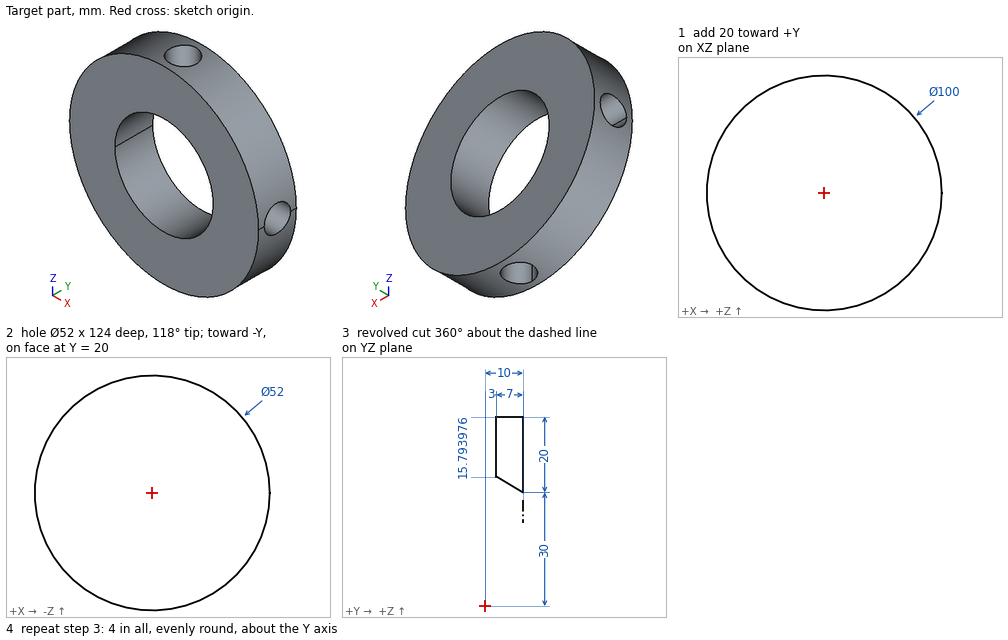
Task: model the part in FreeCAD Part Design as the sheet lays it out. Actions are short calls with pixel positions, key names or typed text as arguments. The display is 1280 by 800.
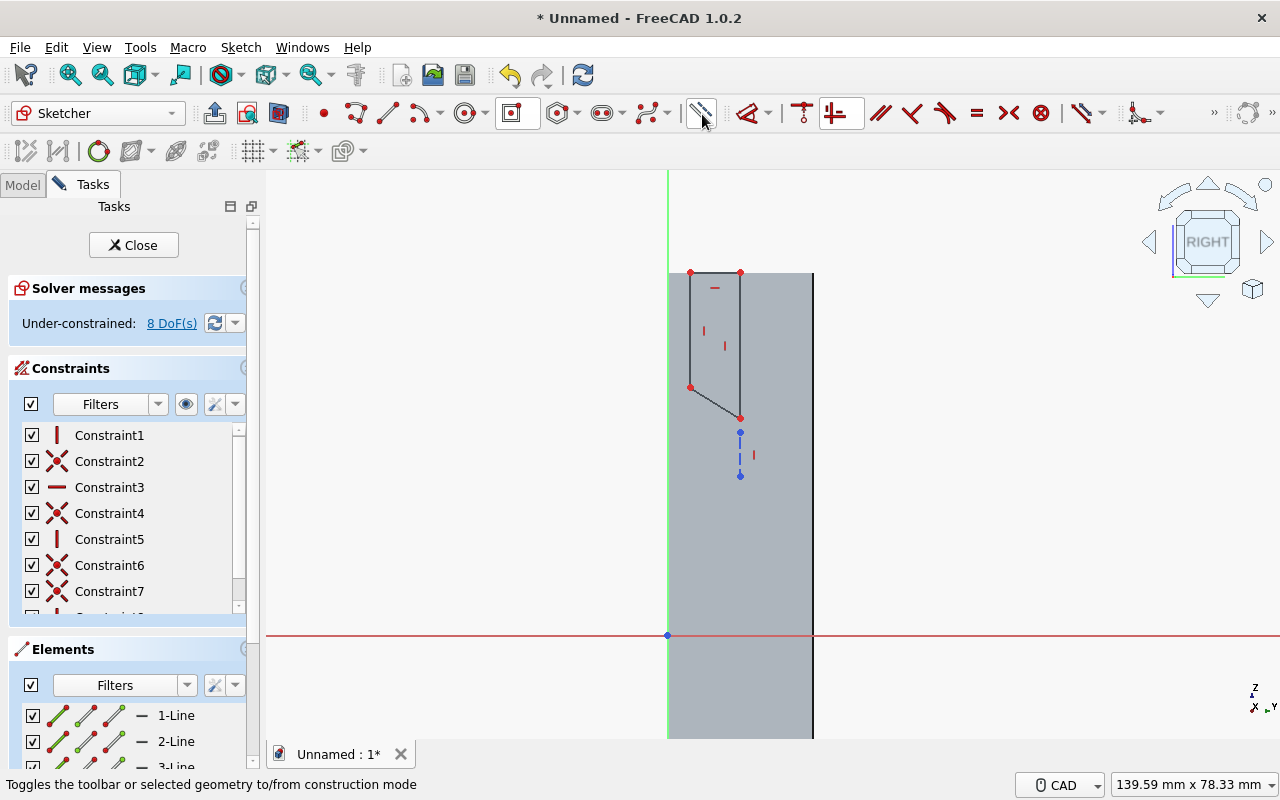
click(725, 273)
click(715, 239)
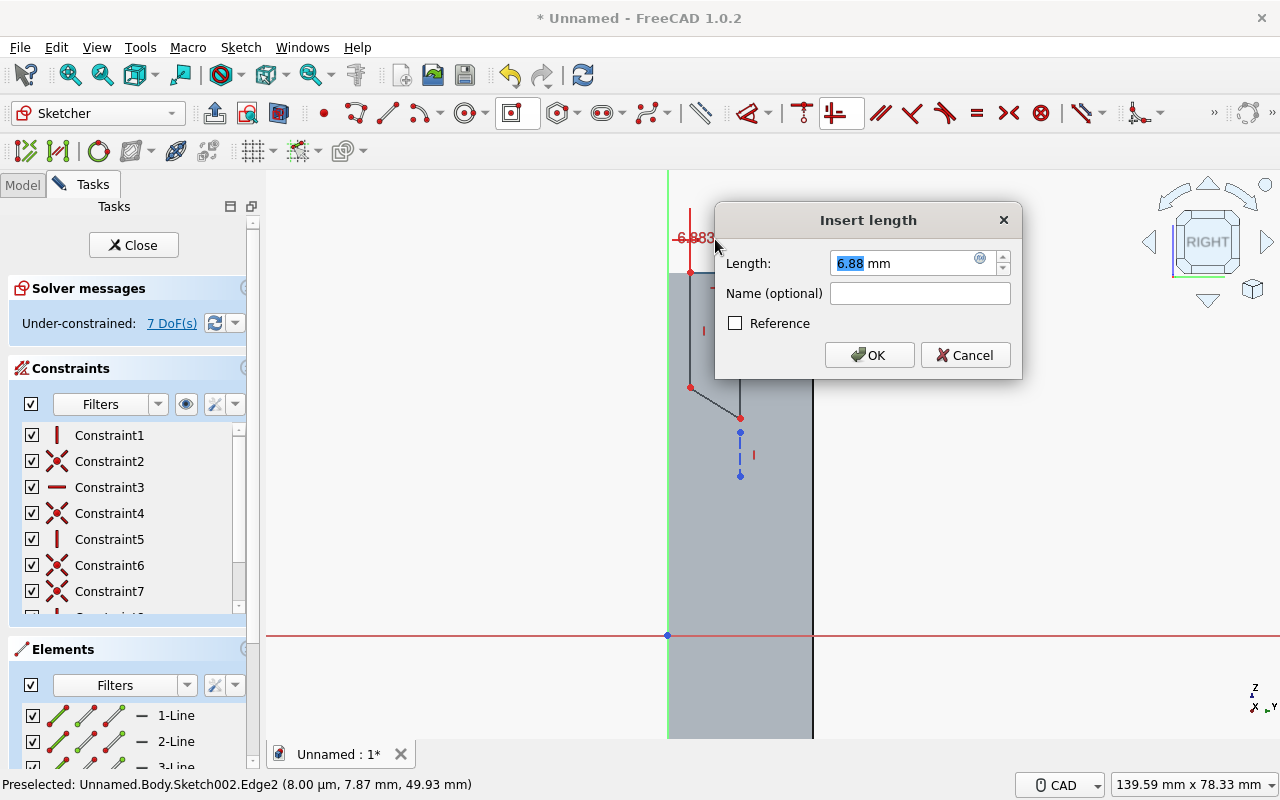
text(7)
key(Return)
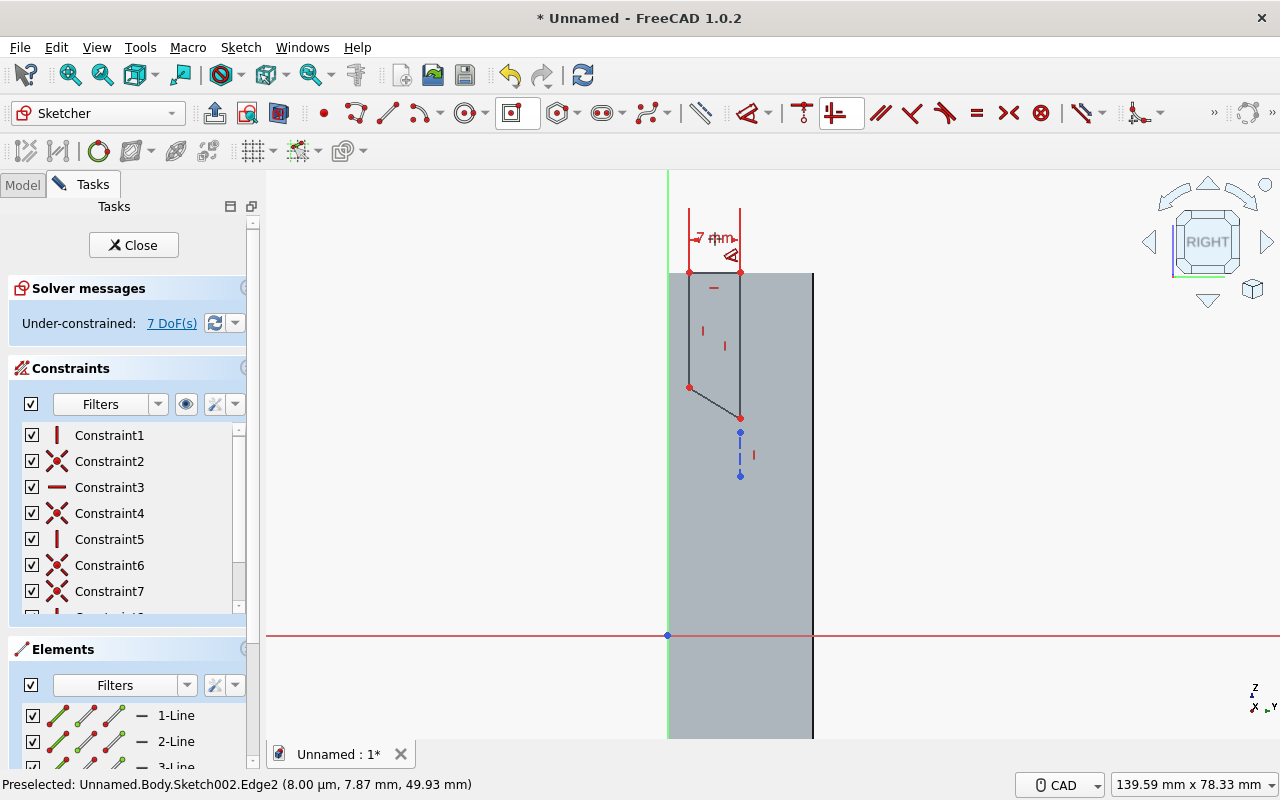
click(740, 375)
click(774, 346)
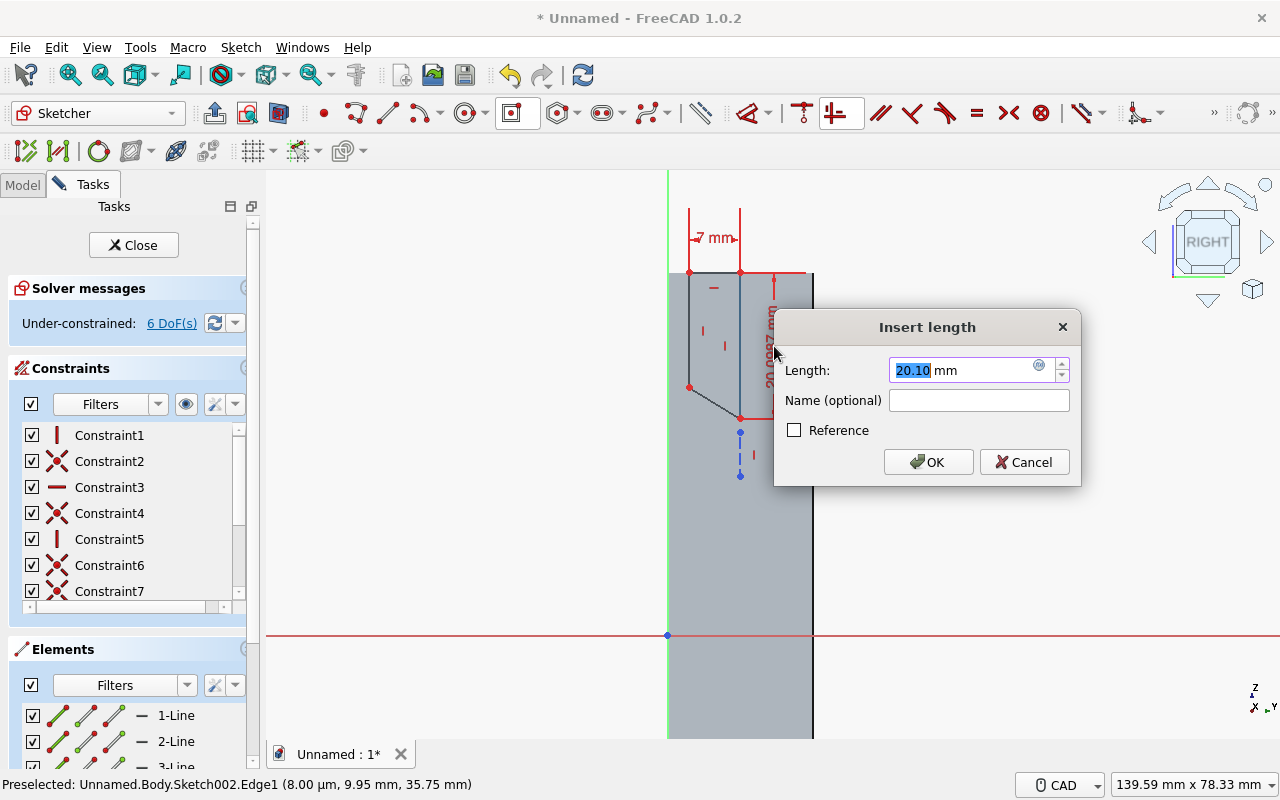
text(20)
key(Return)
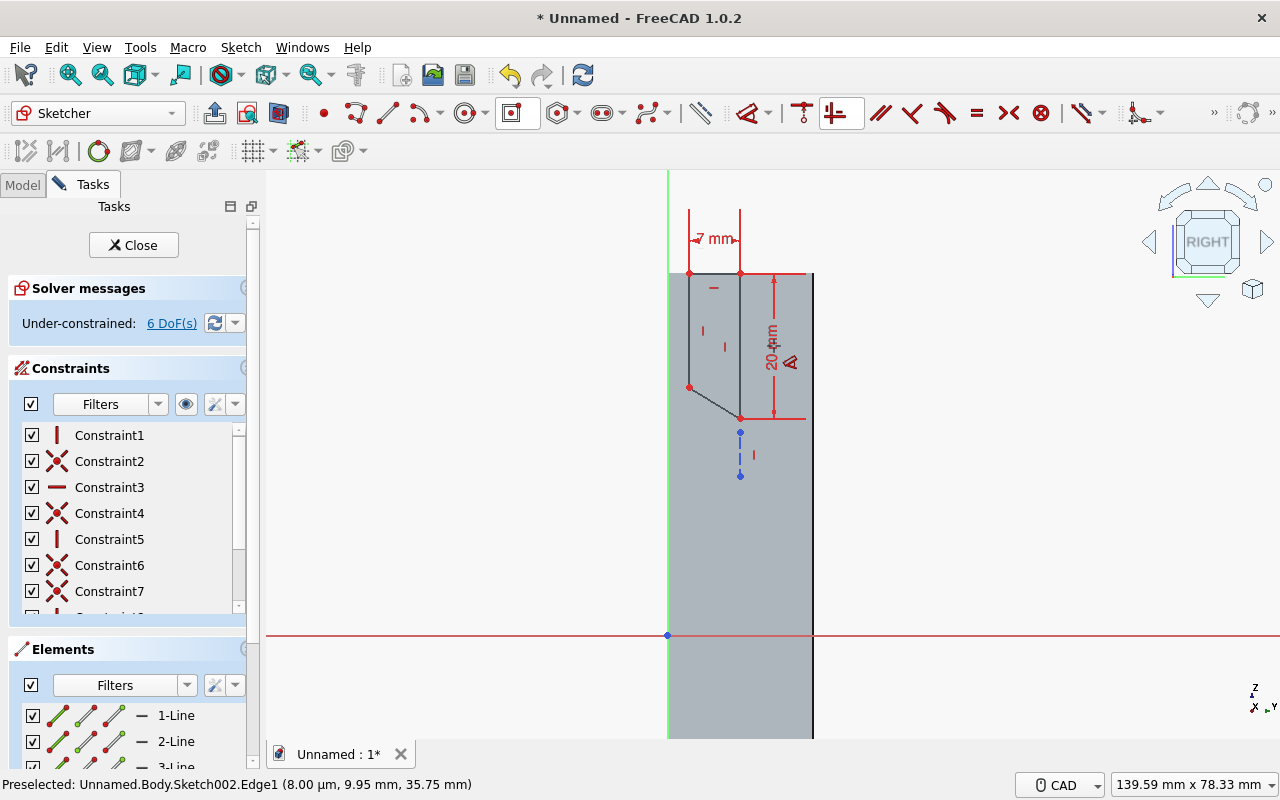
scroll(689, 274, up, 3)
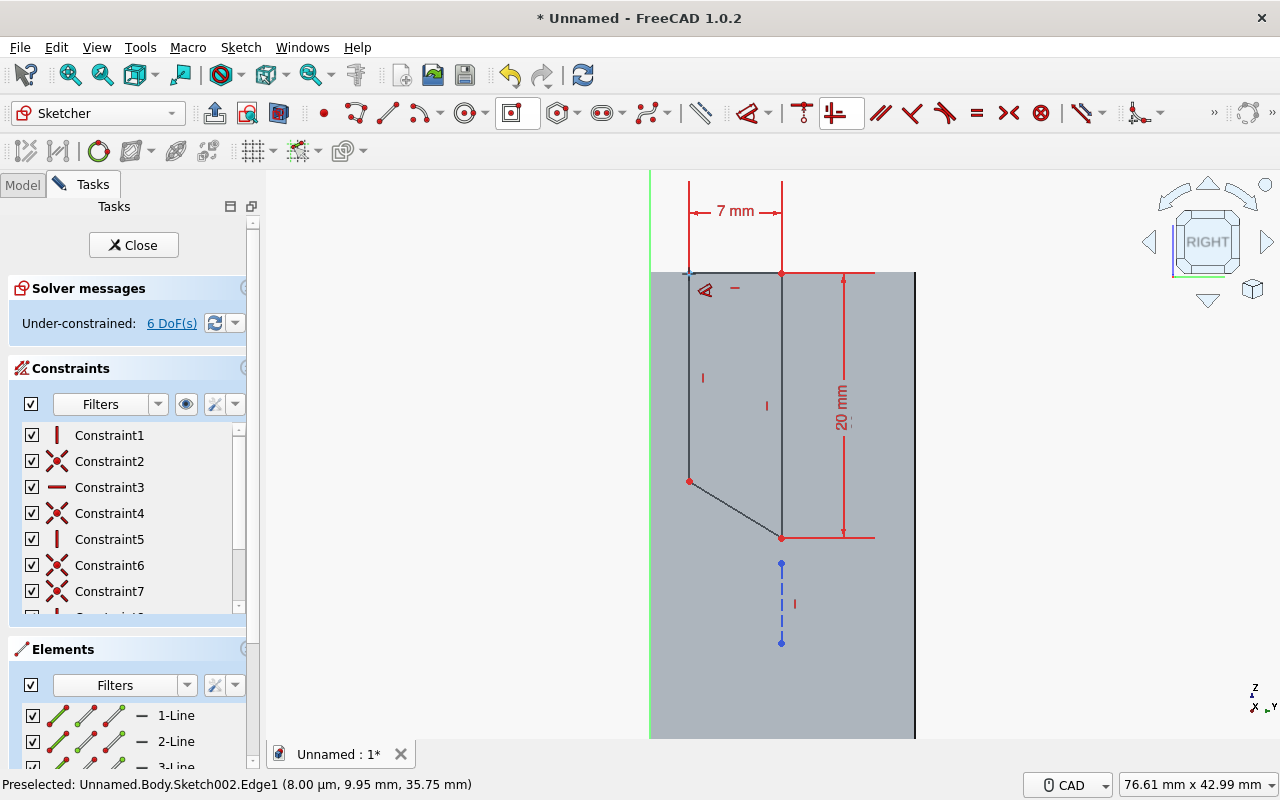
click(689, 273)
click(670, 239)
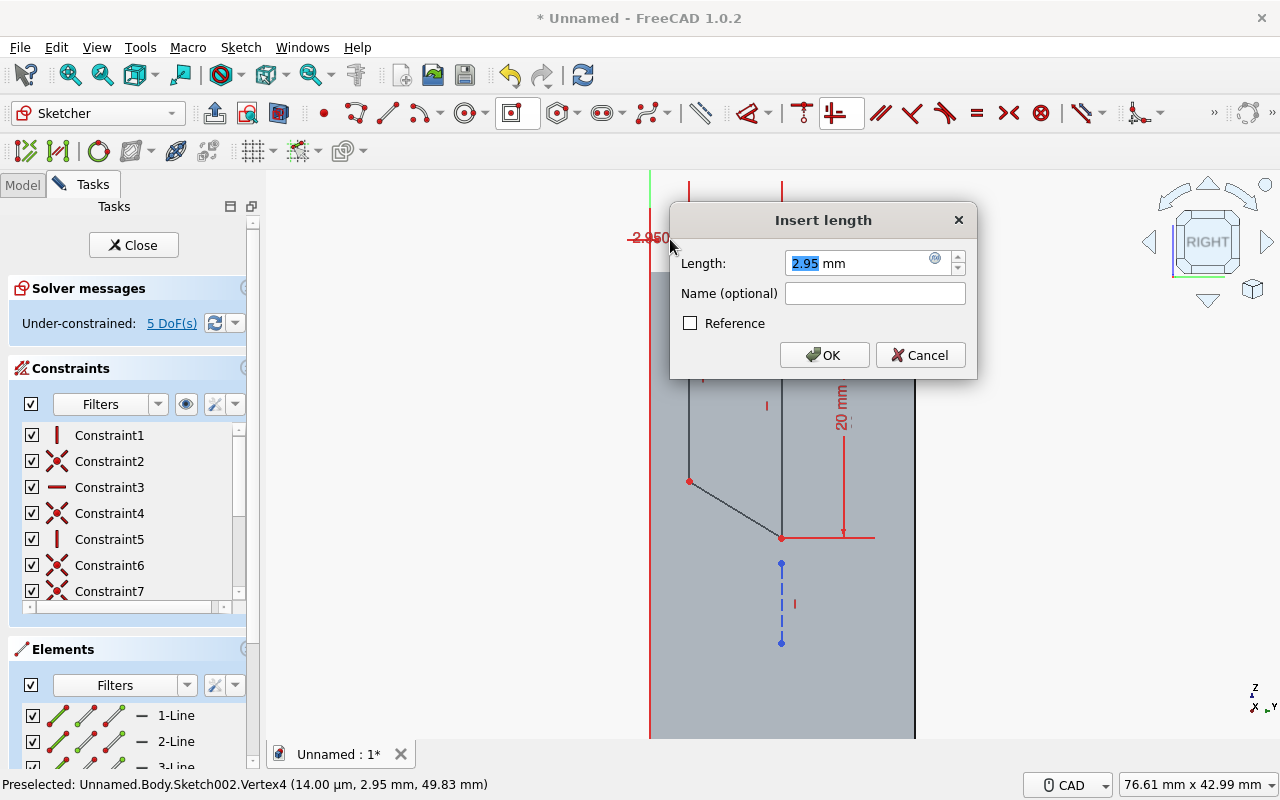
text(3)
key(Return)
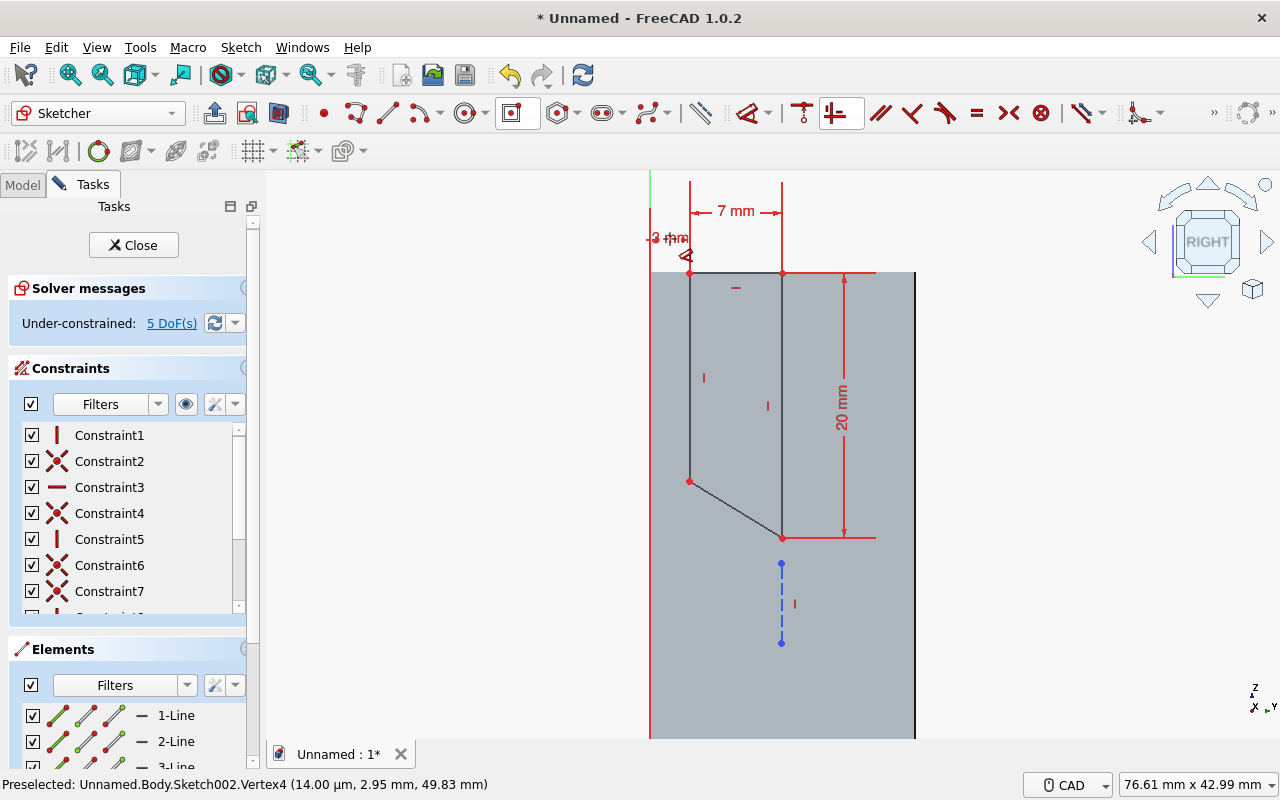
click(782, 538)
click(816, 625)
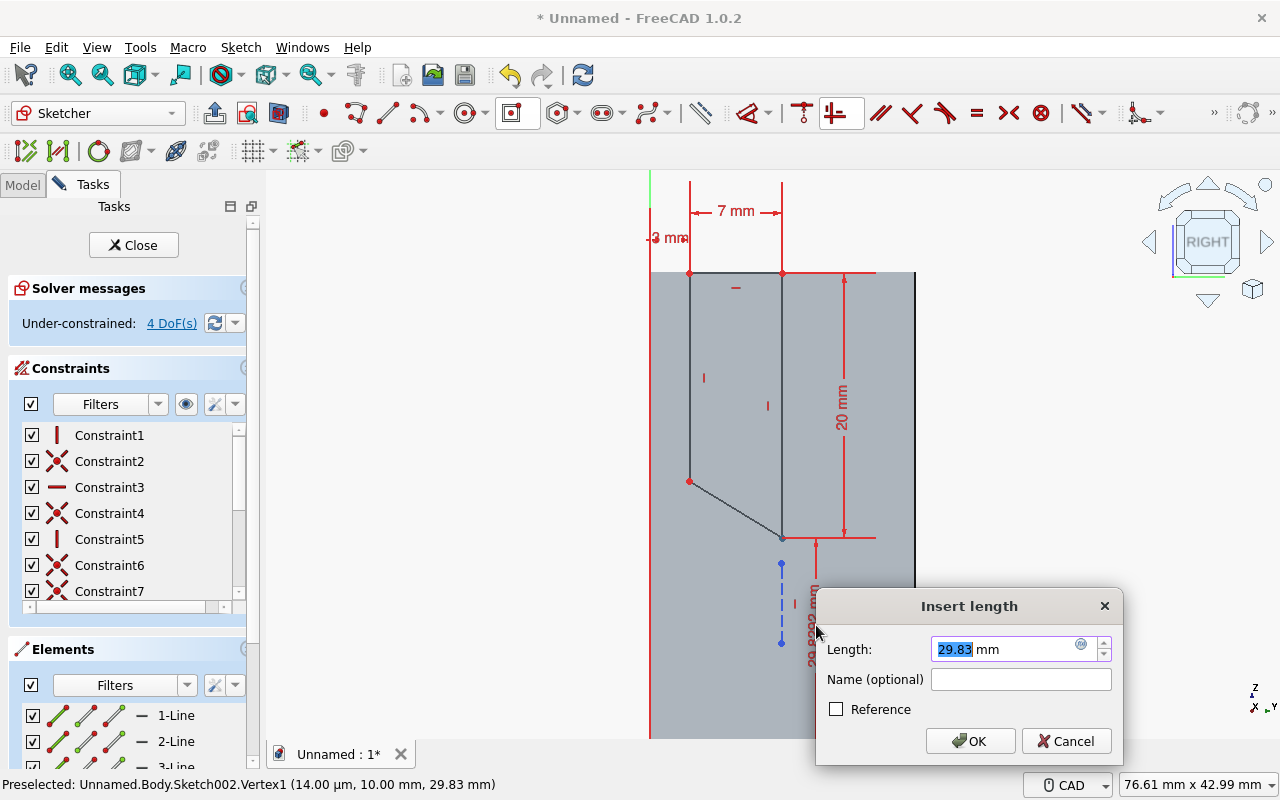
text(30)
key(Return)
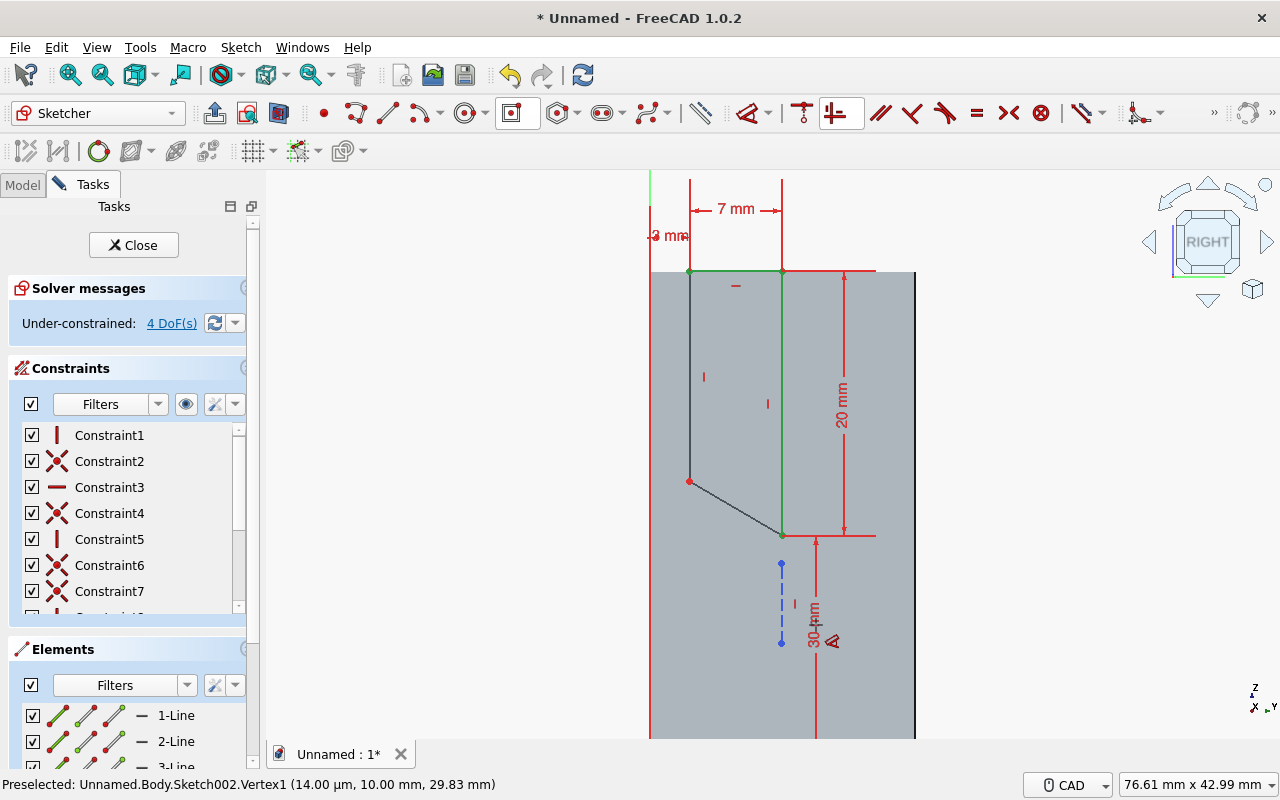
click(782, 564)
click(716, 530)